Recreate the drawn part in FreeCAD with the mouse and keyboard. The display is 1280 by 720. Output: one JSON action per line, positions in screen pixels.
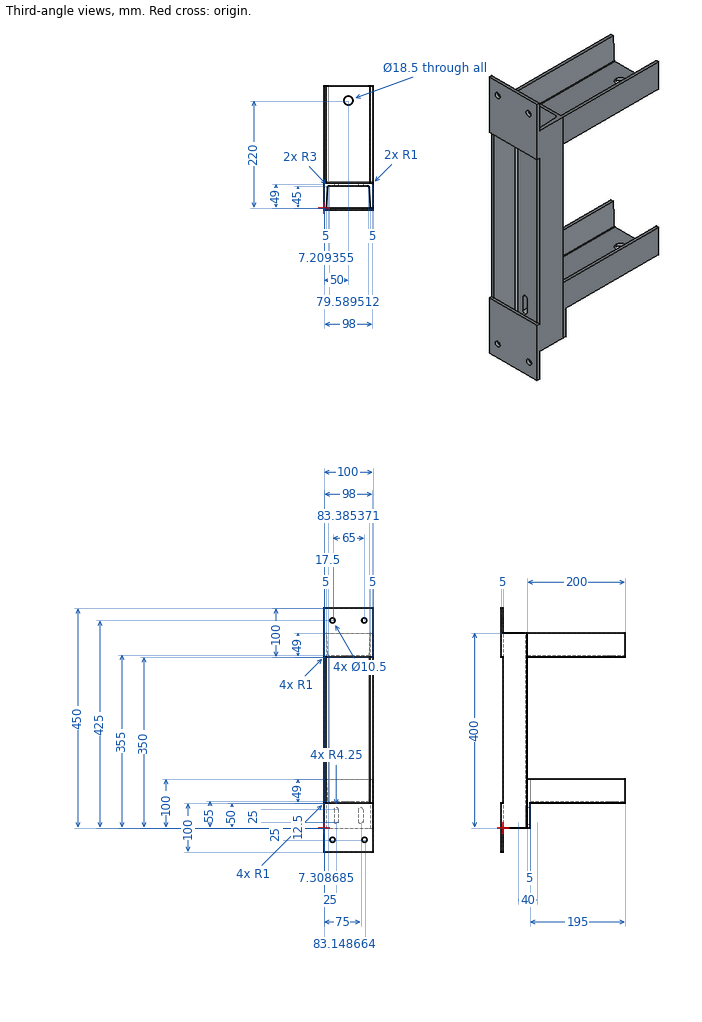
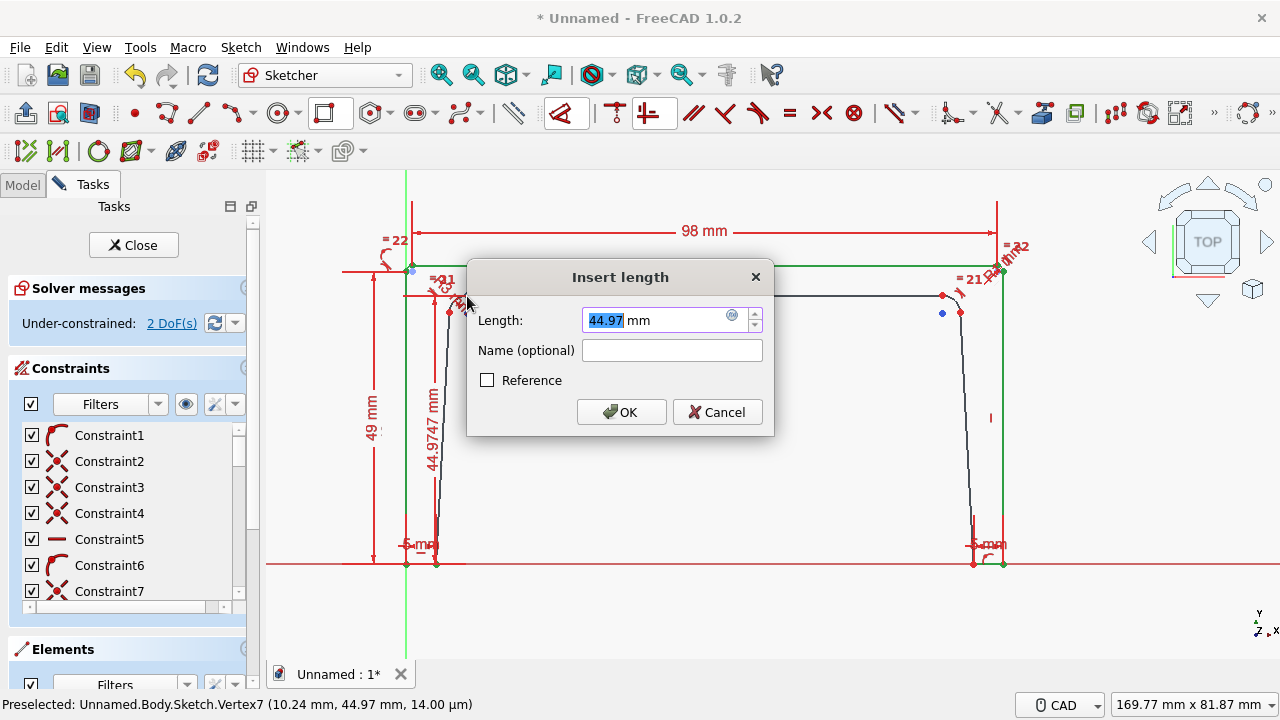
{"action": "type", "text": "45"}
{"action": "key", "text": "Return"}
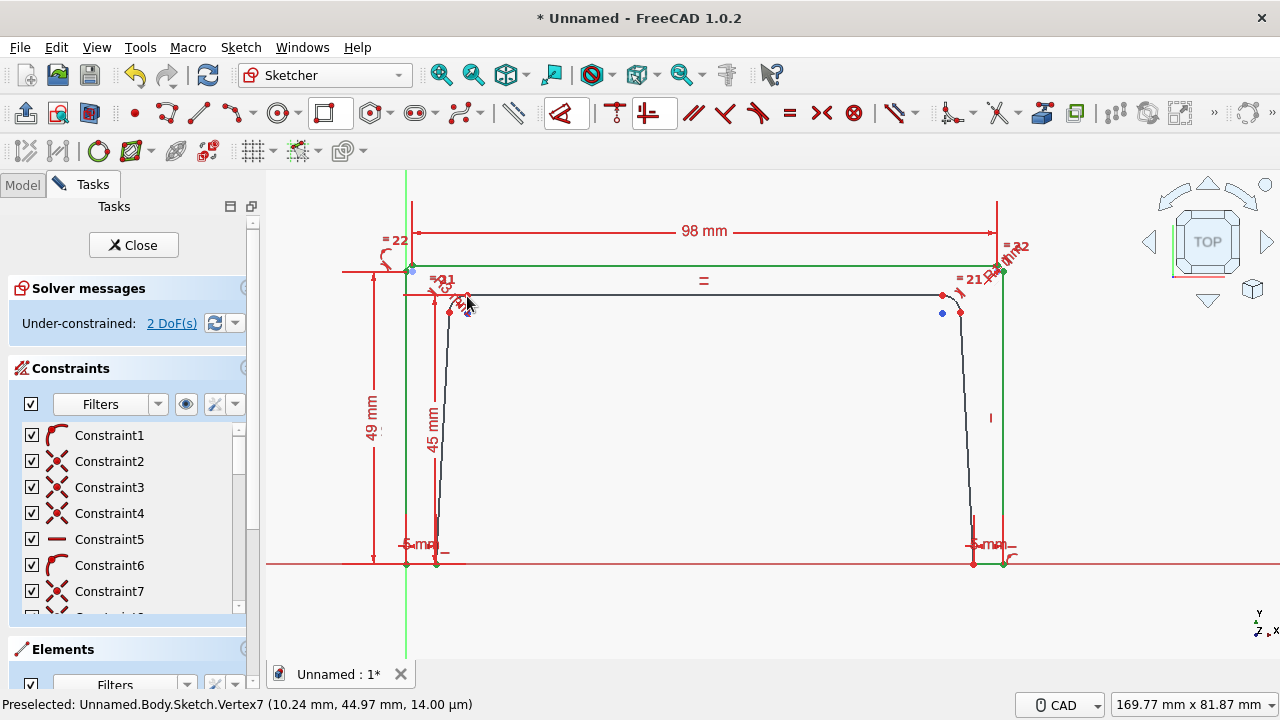
{"action": "left_click", "coordinate": [610, 295]}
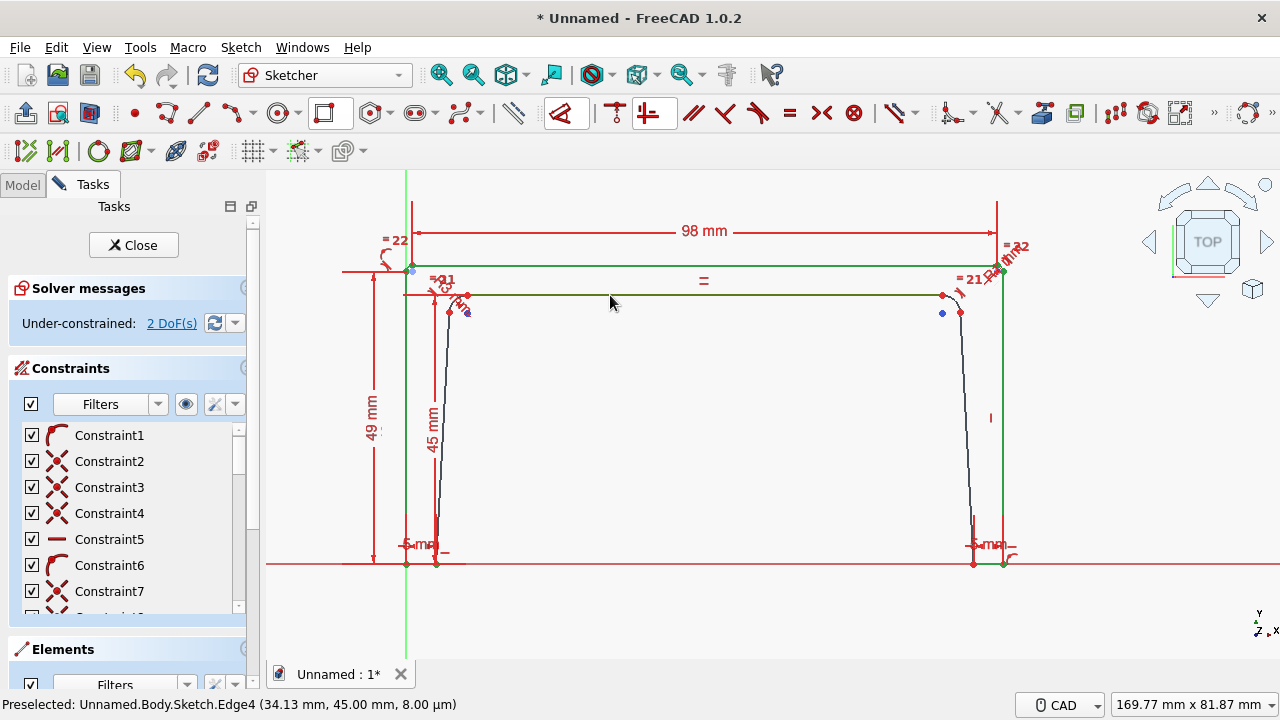
{"action": "key", "text": "l"}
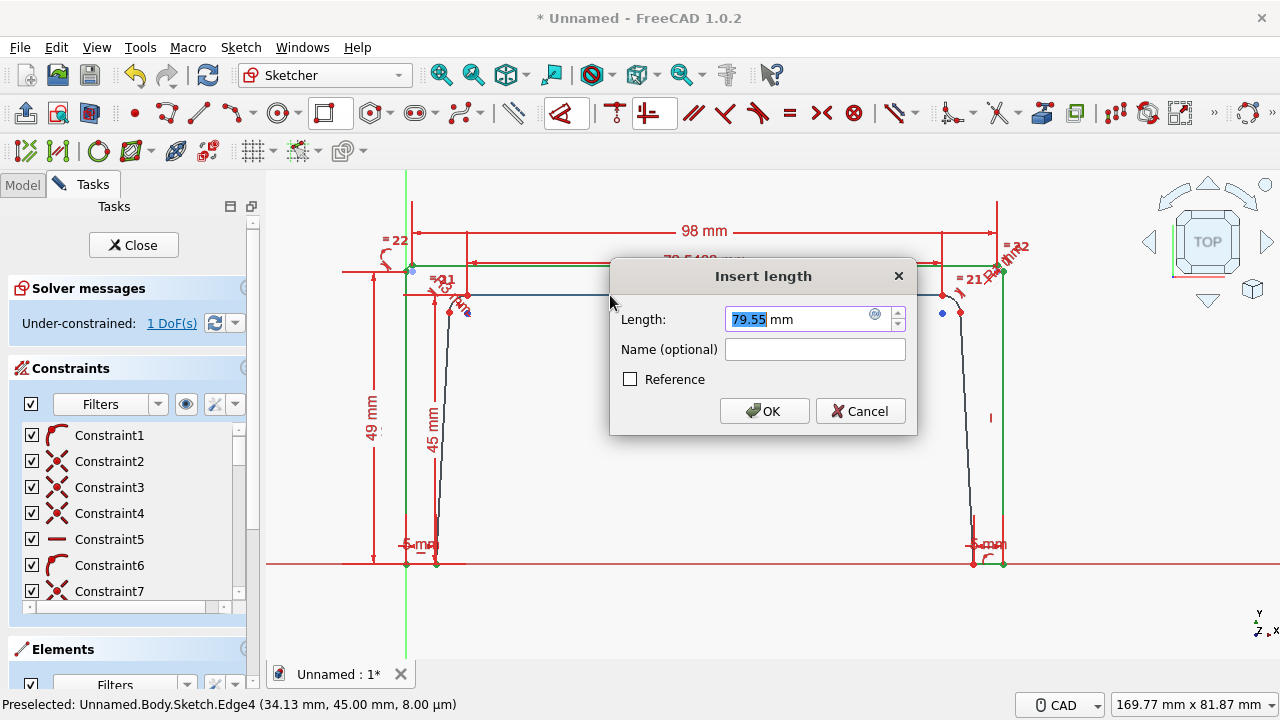
{"action": "type", "text": "79.589512"}
{"action": "key", "text": "Return"}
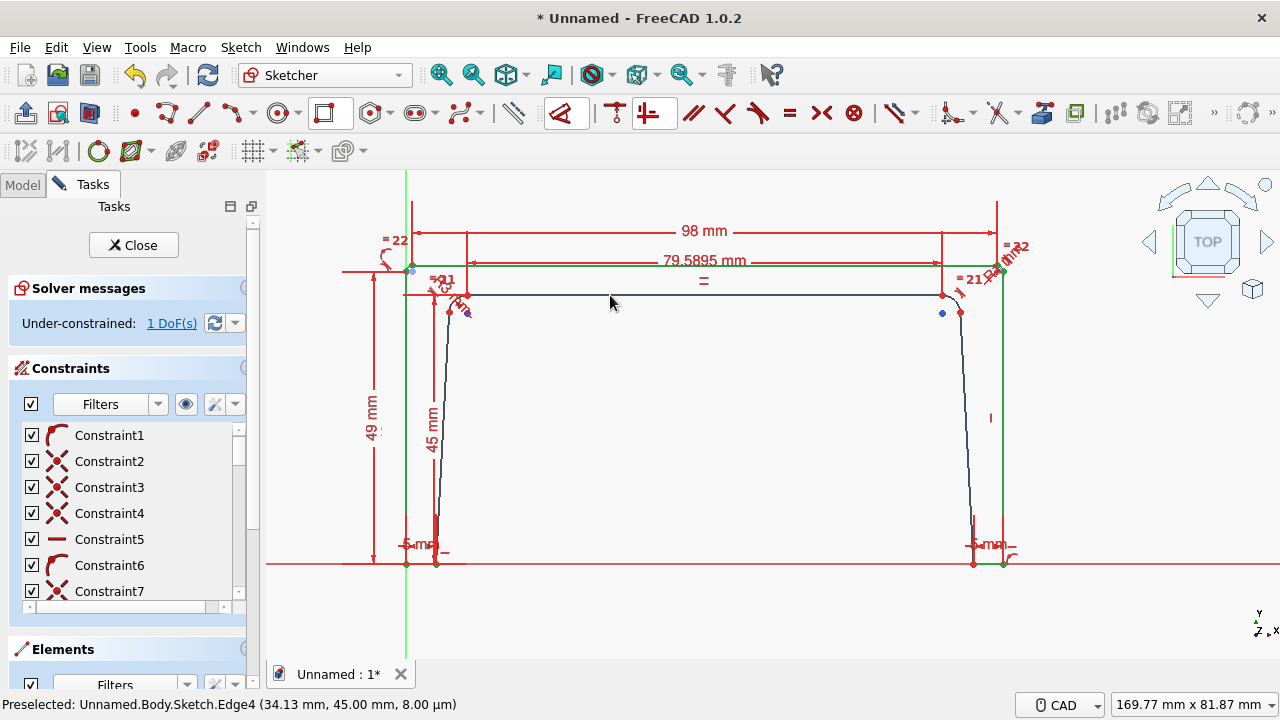
{"action": "left_click", "coordinate": [449, 312]}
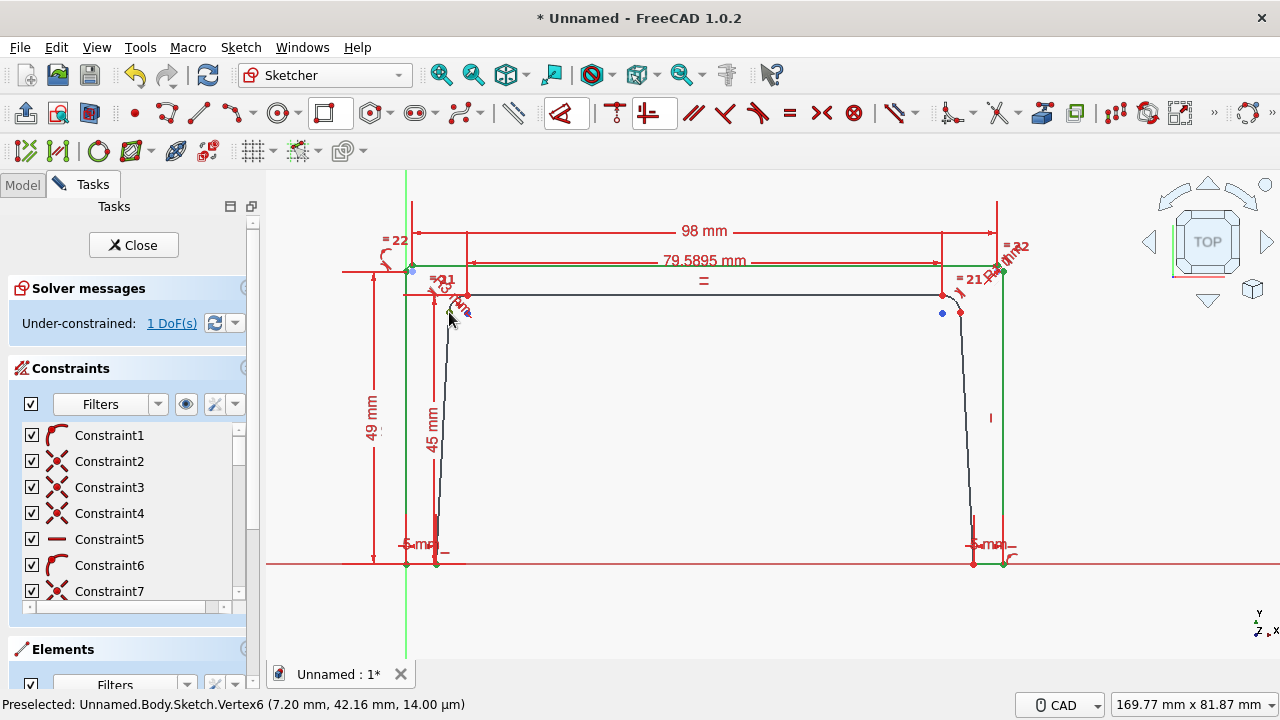
{"action": "key", "text": "l"}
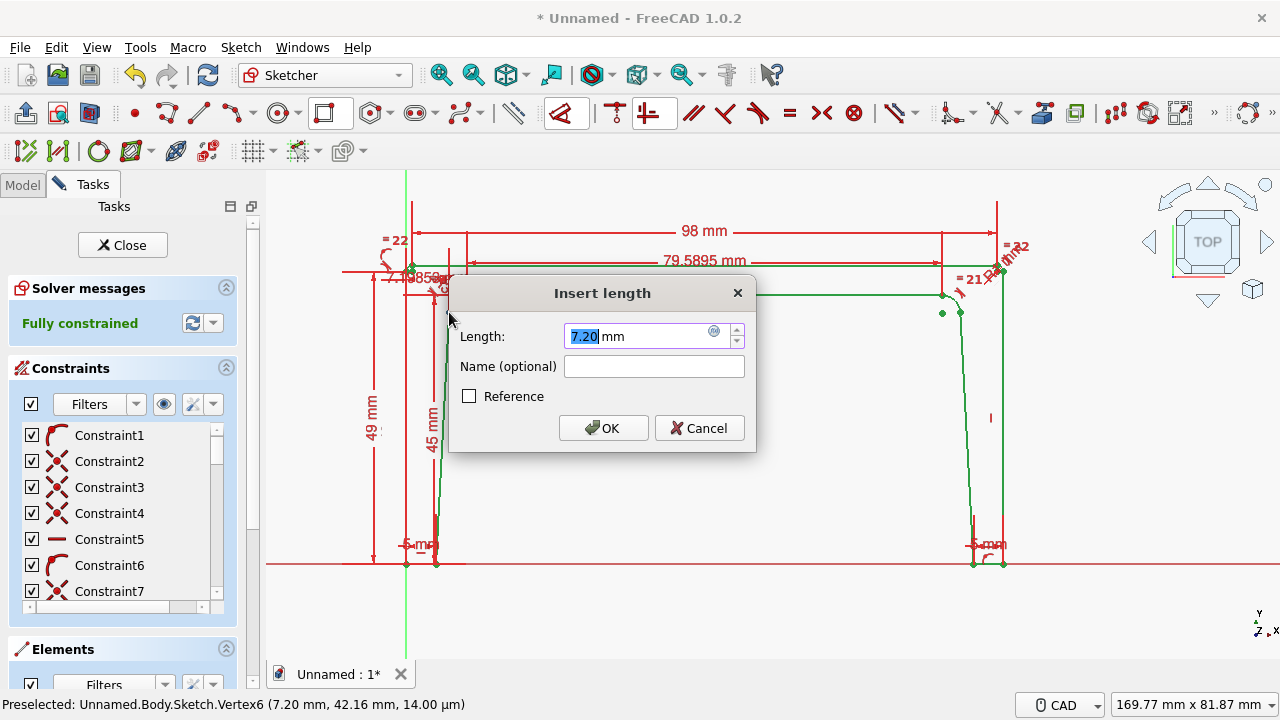
{"action": "type", "text": "7.209355"}
{"action": "key", "text": "Return"}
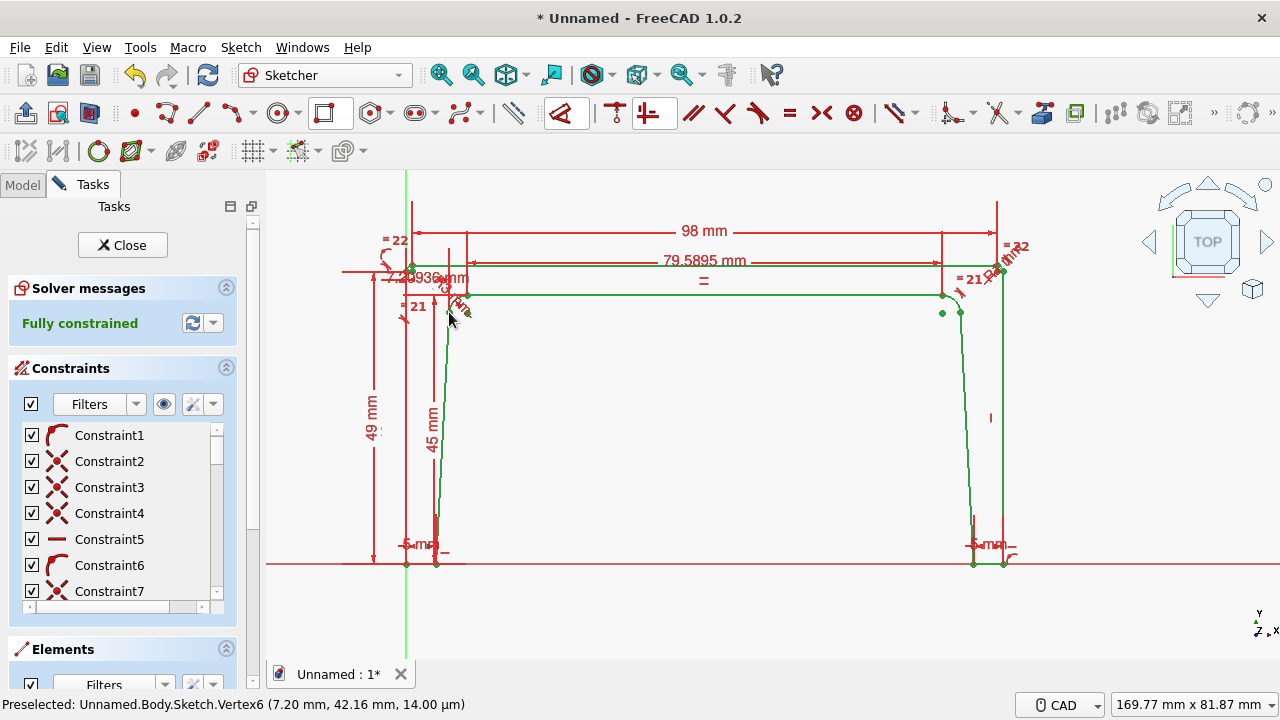
{"action": "left_click", "coordinate": [123, 245]}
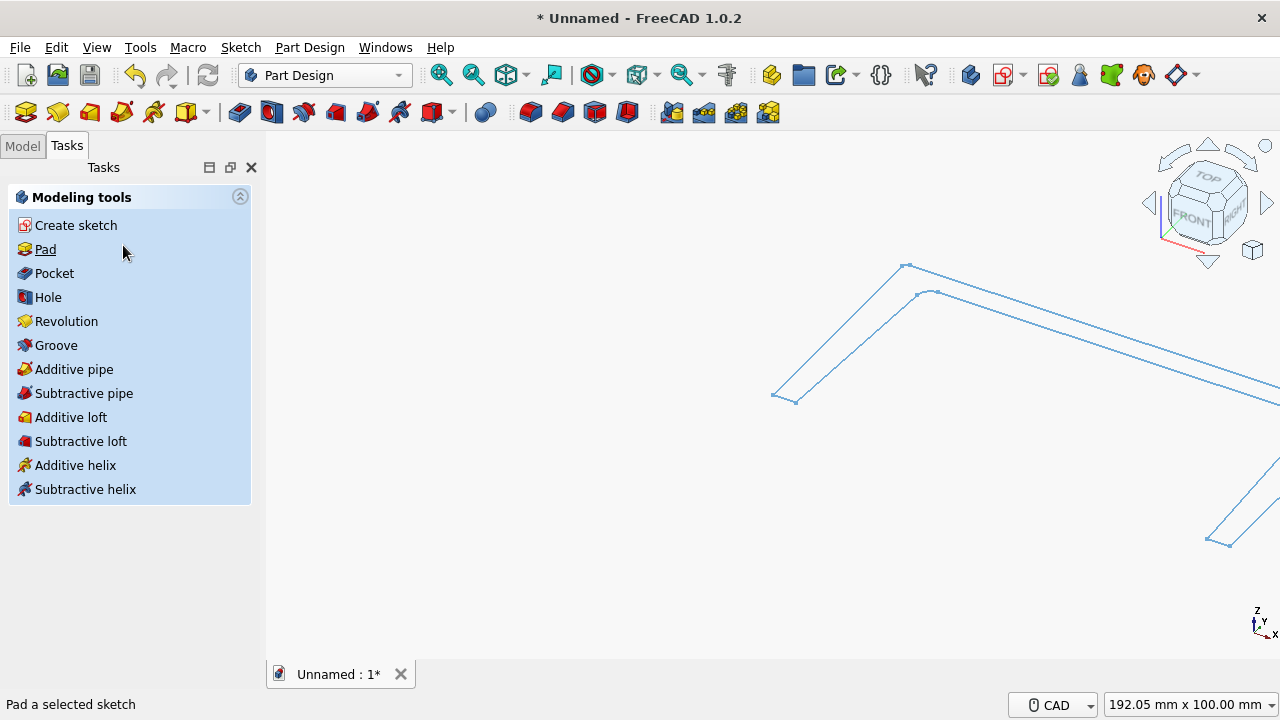
{"action": "left_click", "coordinate": [26, 112]}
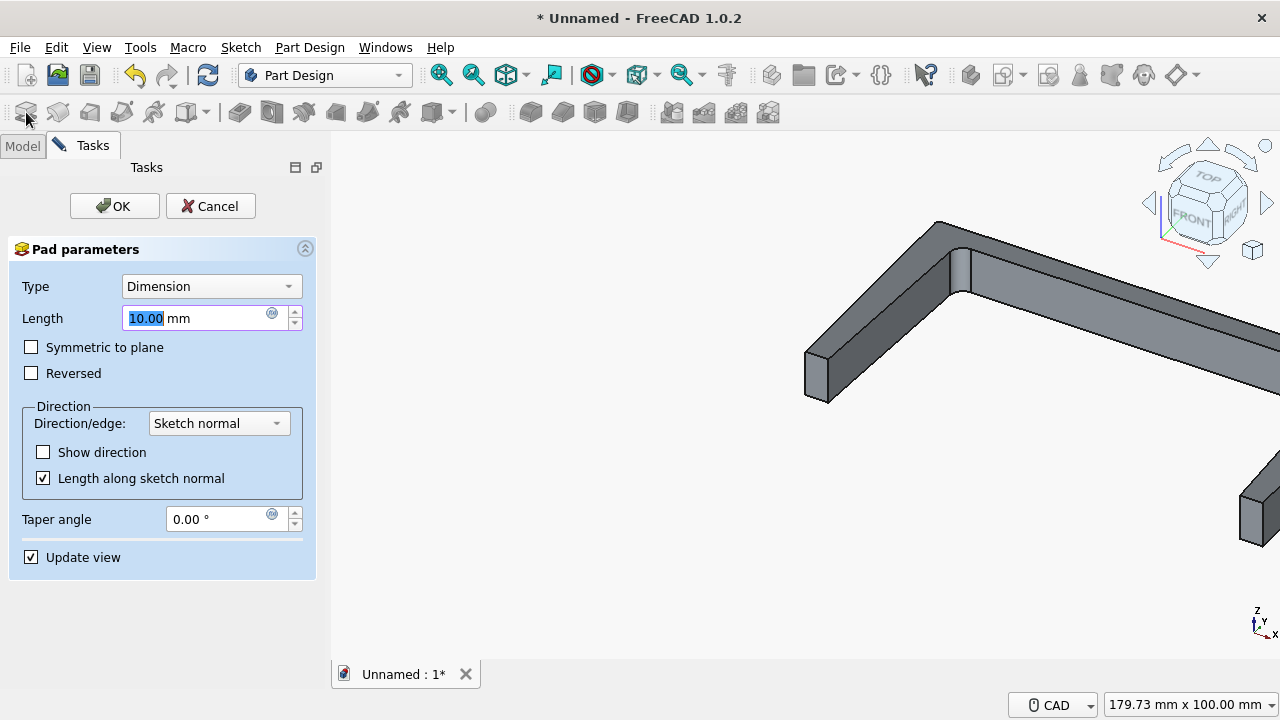
{"action": "type", "text": "400"}
{"action": "key", "text": "Tab"}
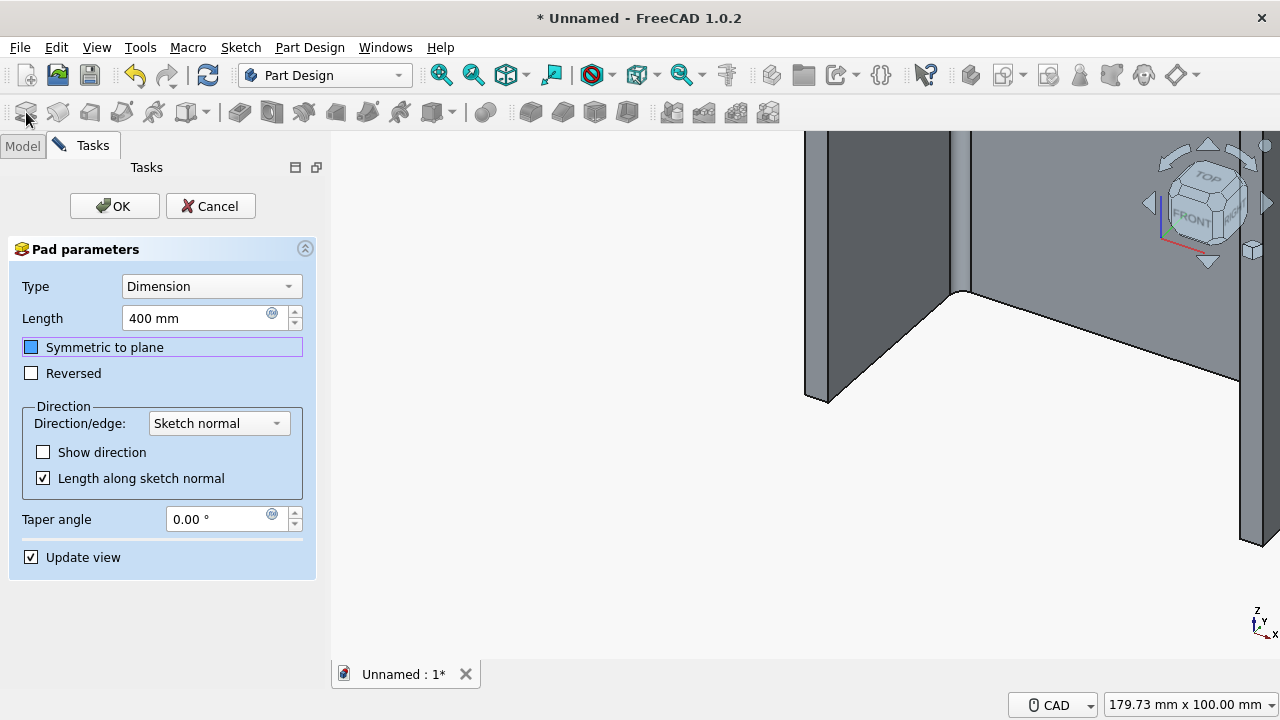
{"action": "left_click", "coordinate": [115, 206]}